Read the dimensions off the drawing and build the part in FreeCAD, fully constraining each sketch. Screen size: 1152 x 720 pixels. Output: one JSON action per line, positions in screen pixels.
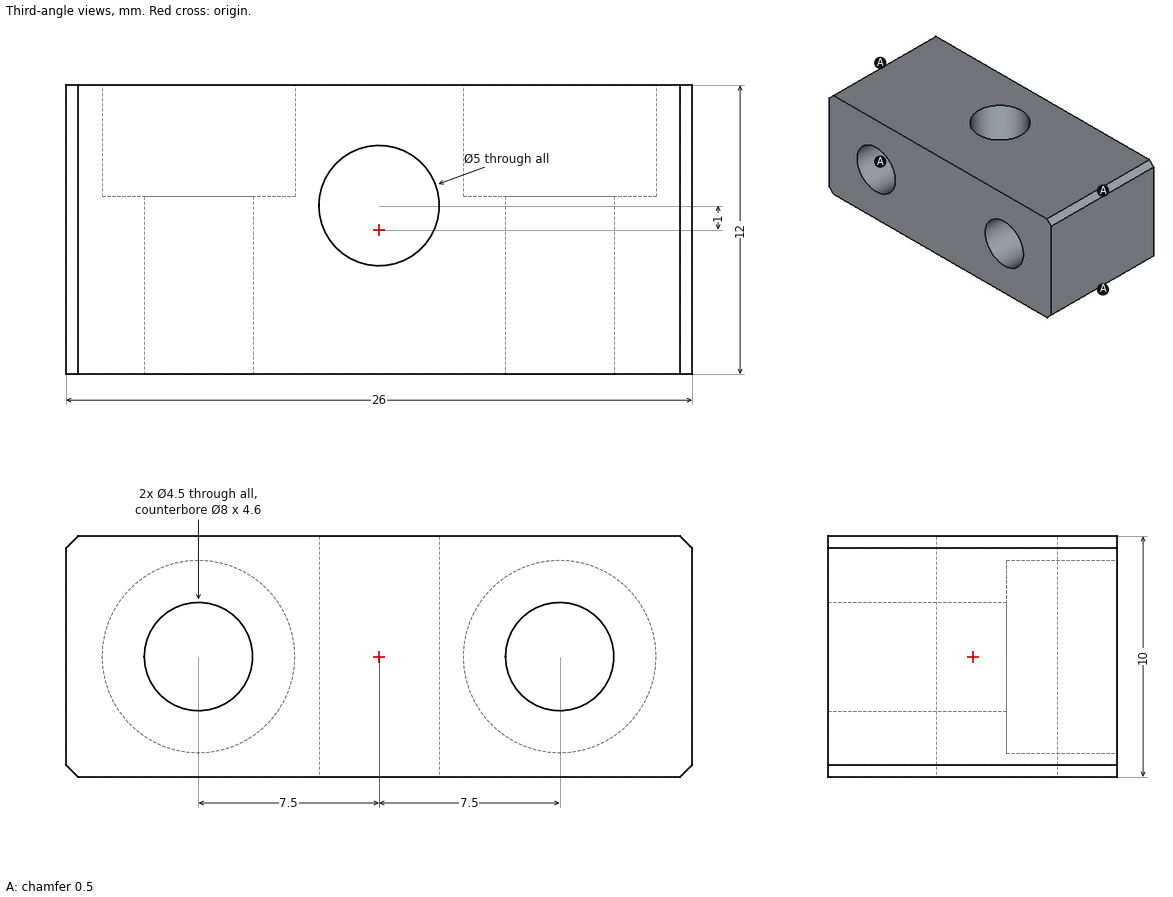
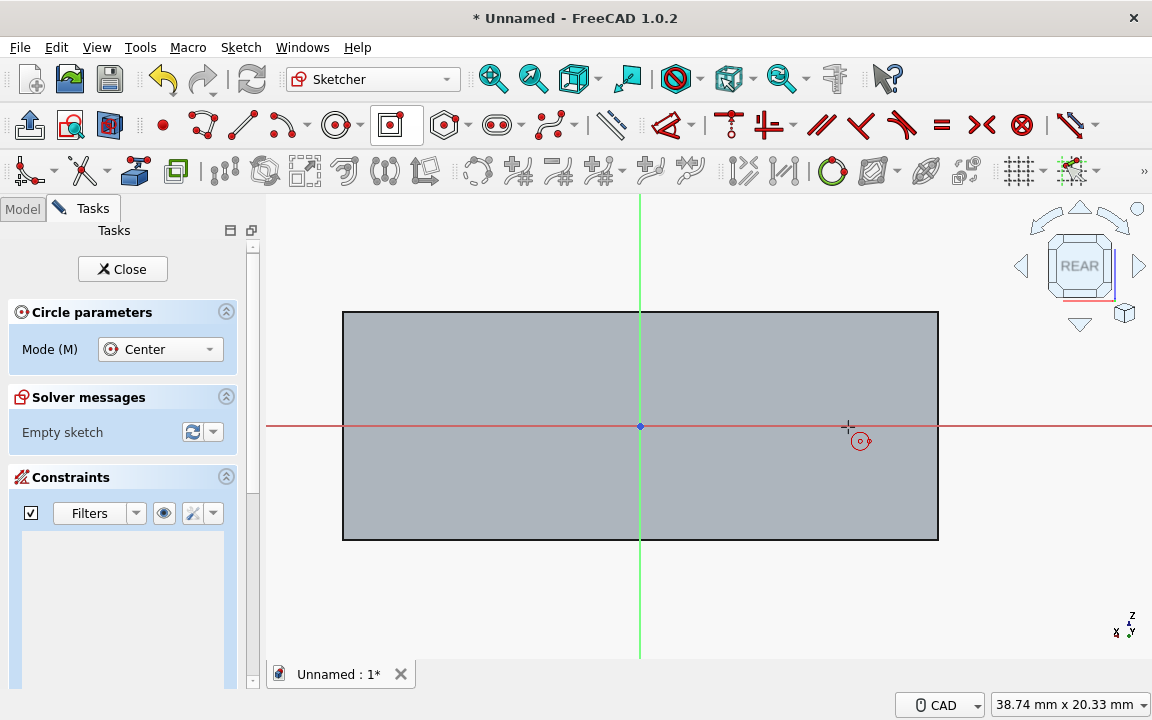
{"action": "left_click", "coordinate": [812, 426]}
{"action": "left_click", "coordinate": [848, 390]}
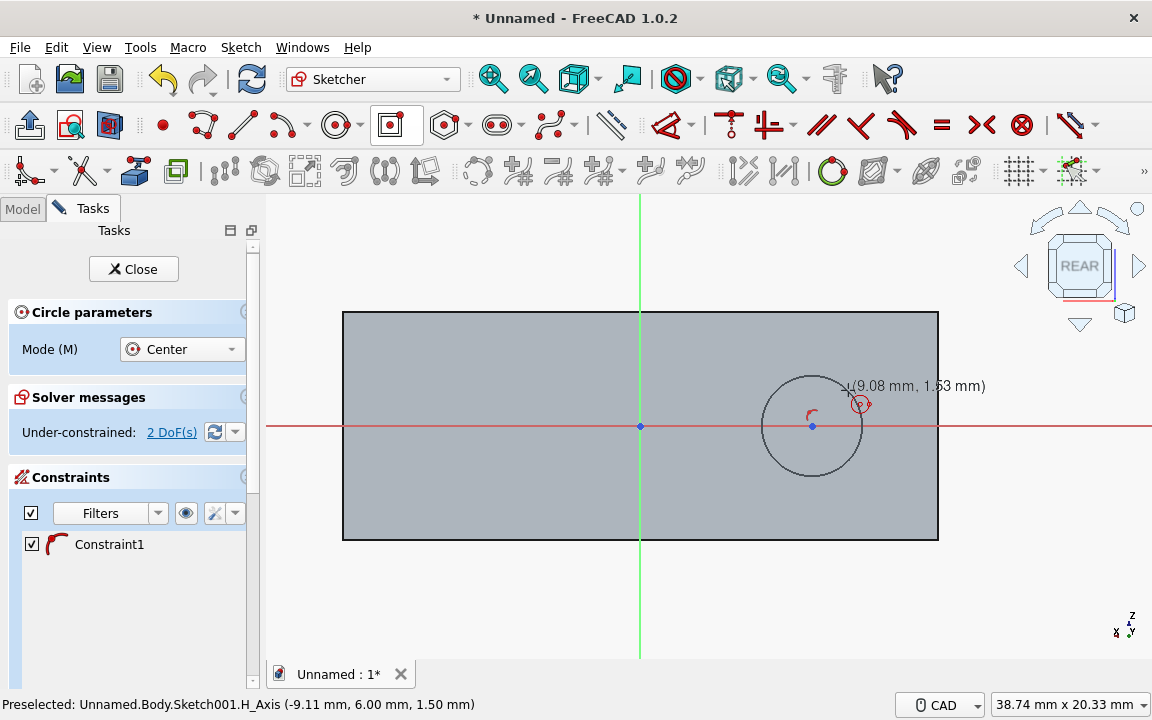
{"action": "left_click", "coordinate": [469, 426]}
{"action": "left_click", "coordinate": [505, 390]}
{"action": "key", "text": "Escape"}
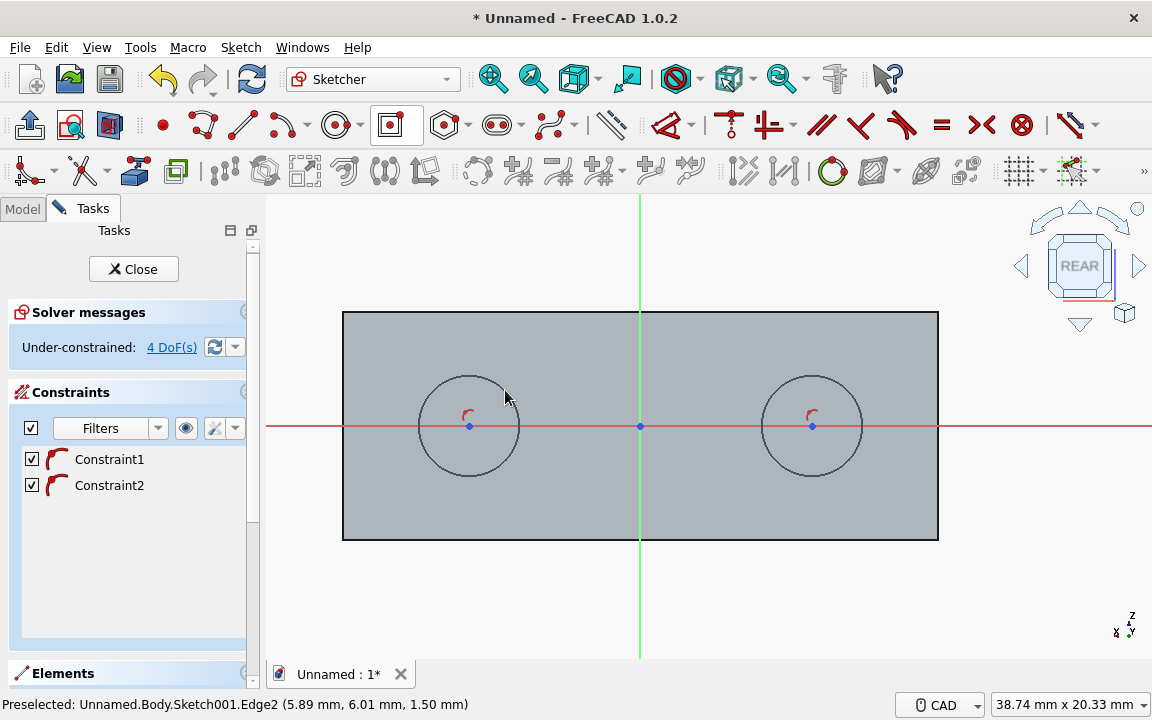
{"action": "left_click", "coordinate": [847, 390]}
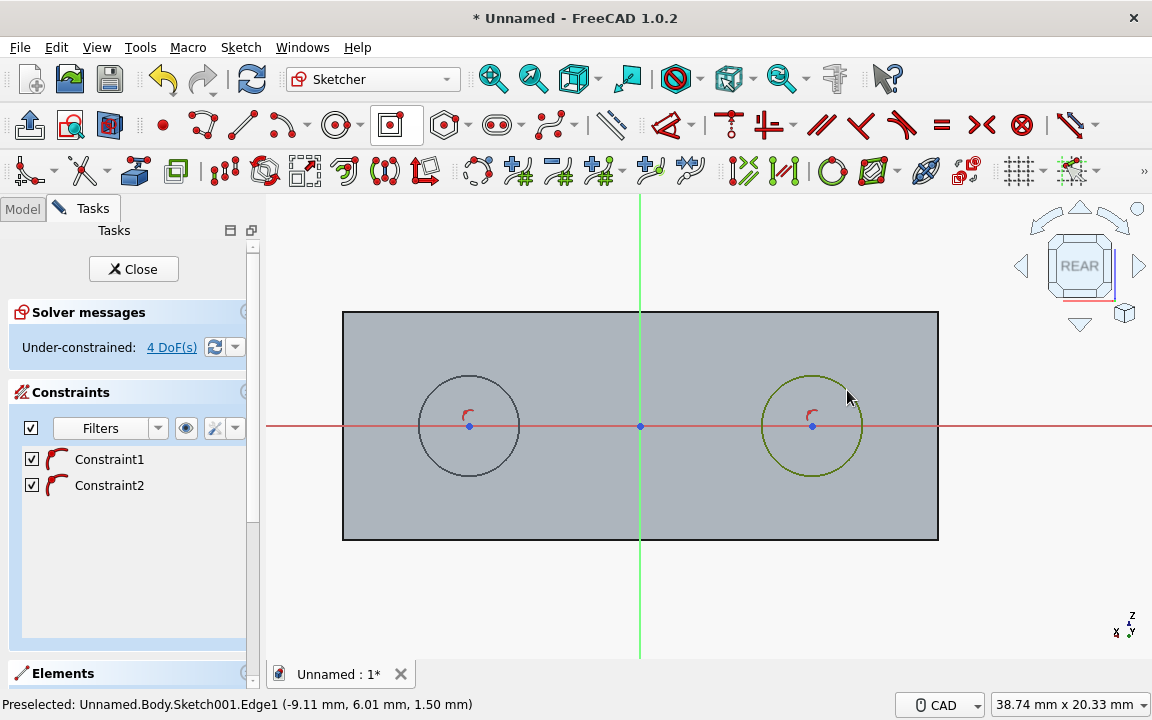
{"action": "left_click", "coordinate": [504, 390]}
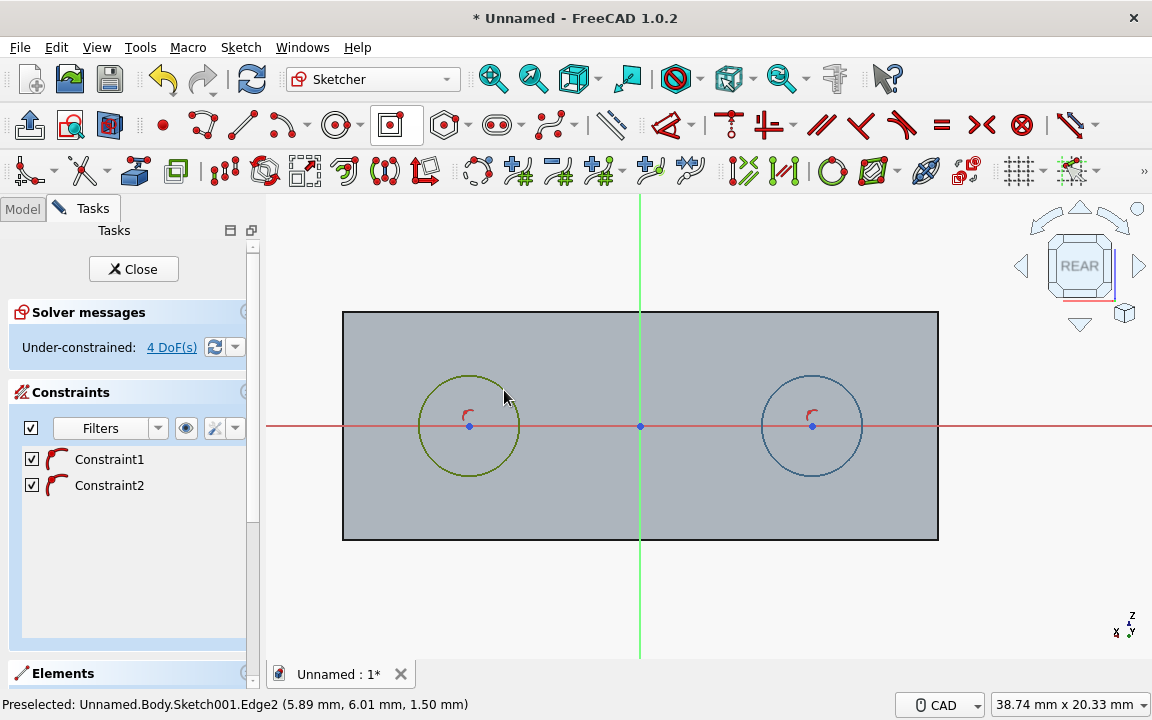
{"action": "key", "text": "e"}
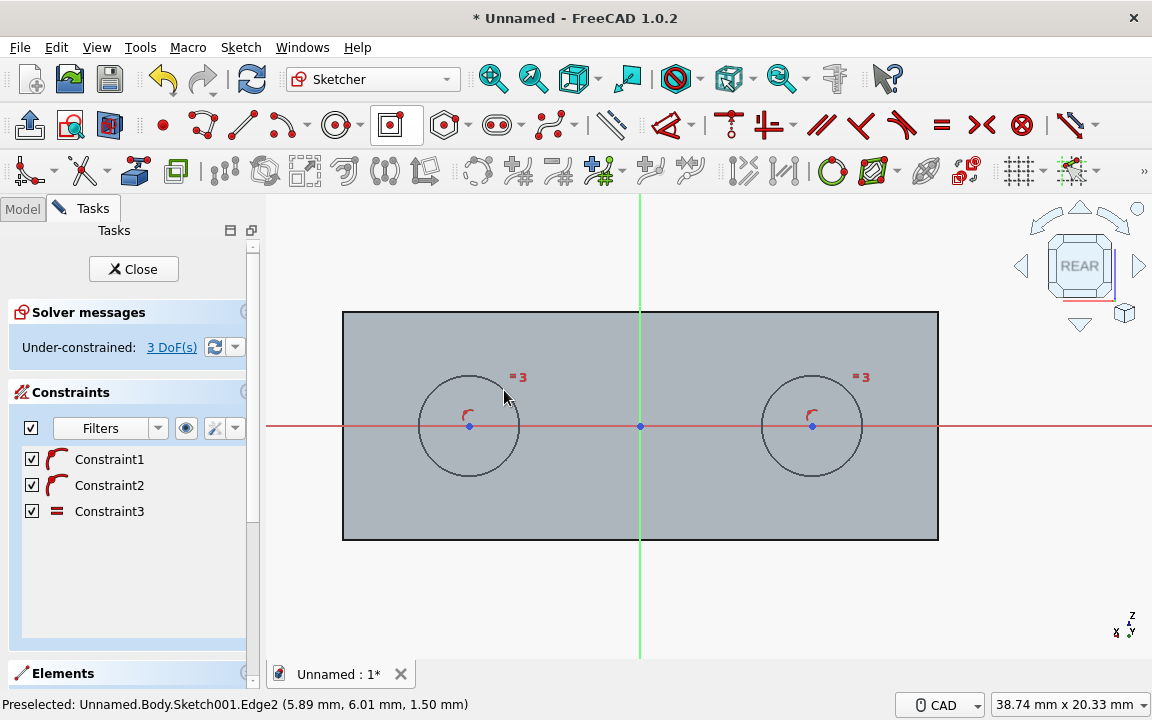
{"action": "left_click", "coordinate": [847, 390]}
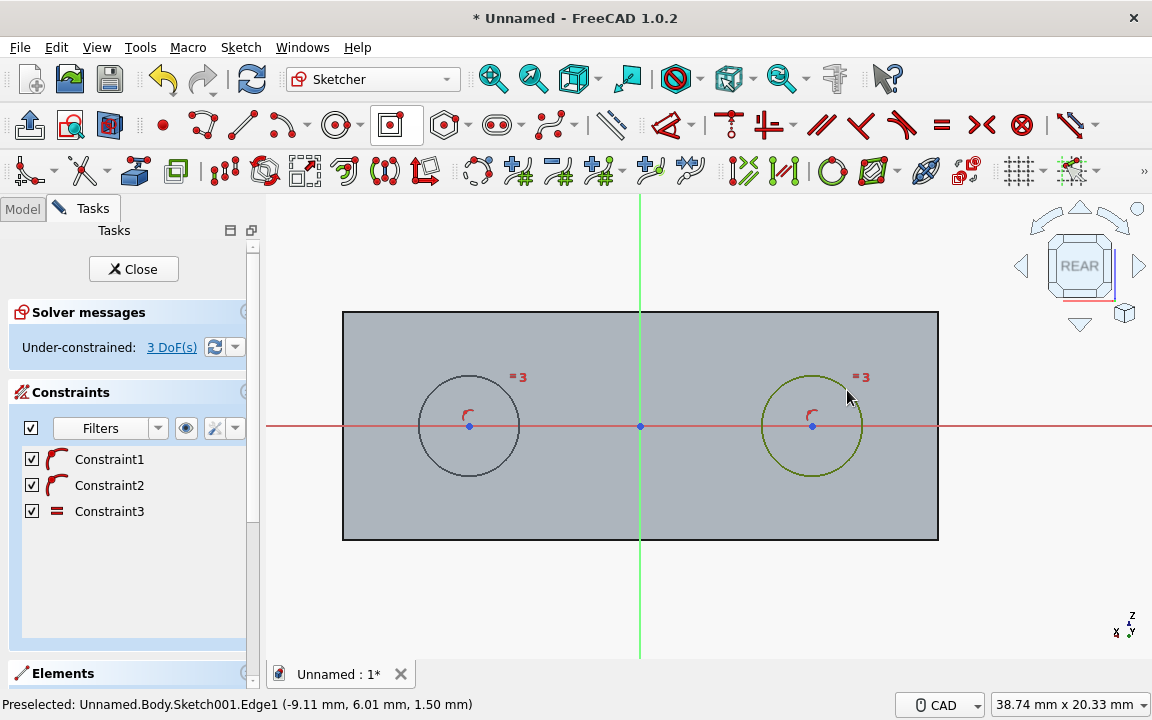
{"action": "key", "text": "k o"}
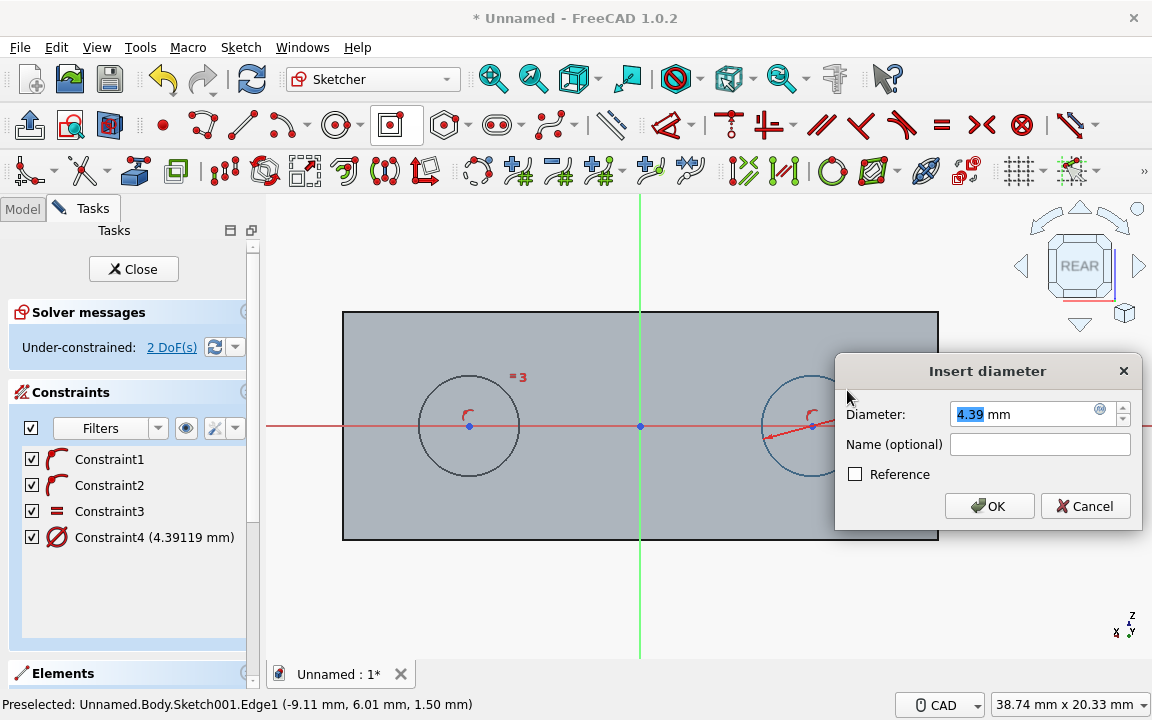
{"action": "type", "text": "4.5"}
{"action": "key", "text": "Return"}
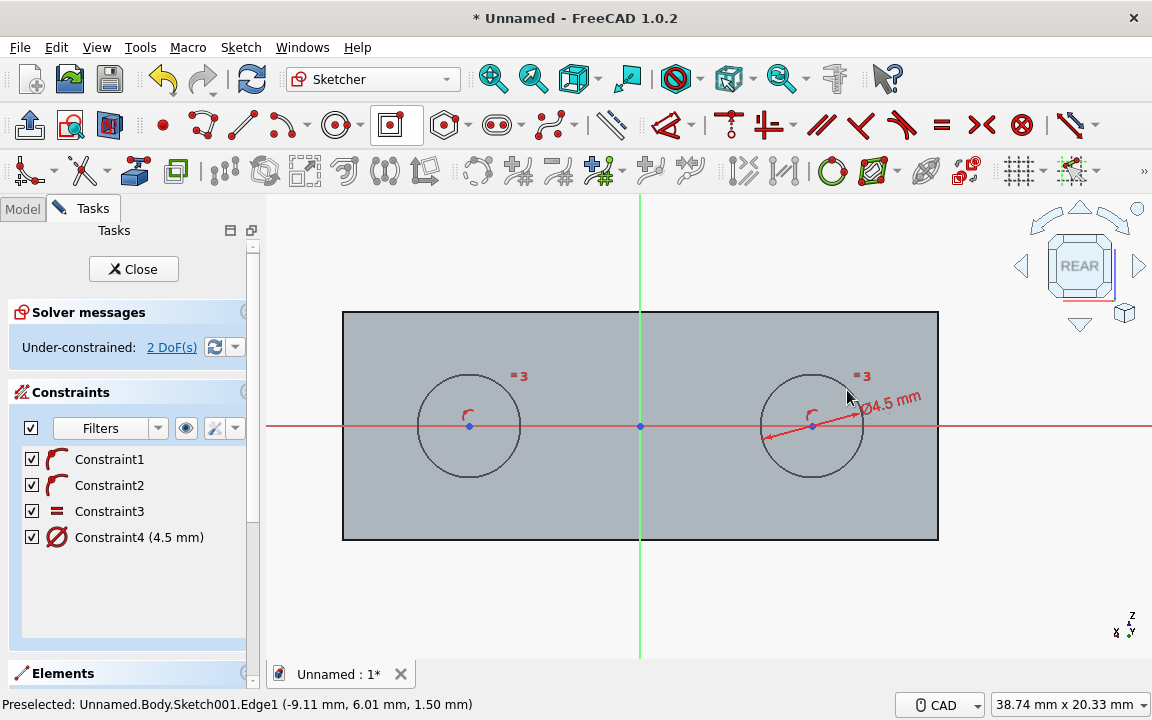
{"action": "left_click", "coordinate": [812, 426]}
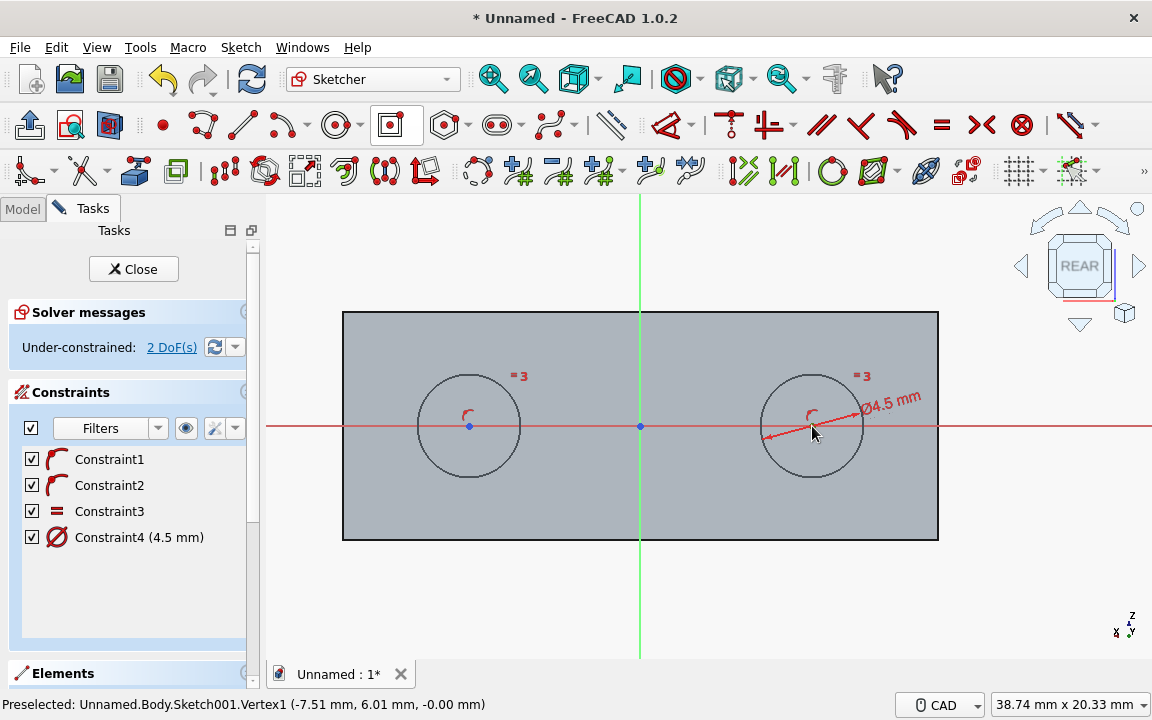
{"action": "key", "text": "l"}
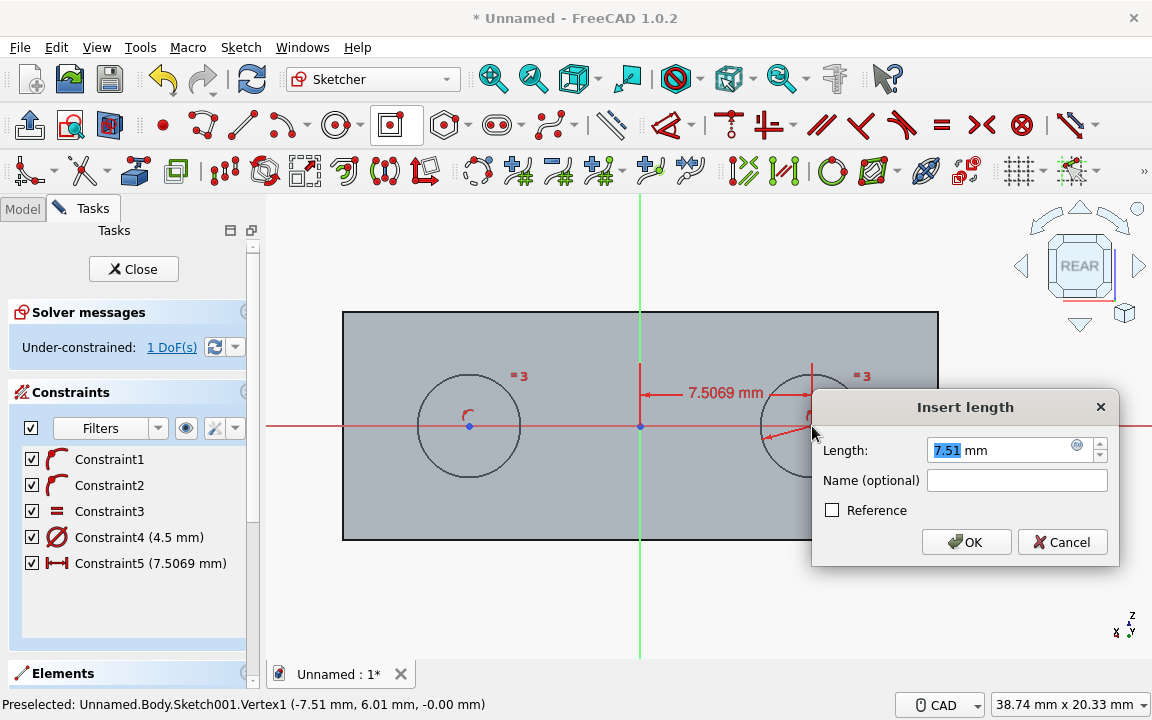
{"action": "type", "text": "7.5"}
{"action": "key", "text": "Return"}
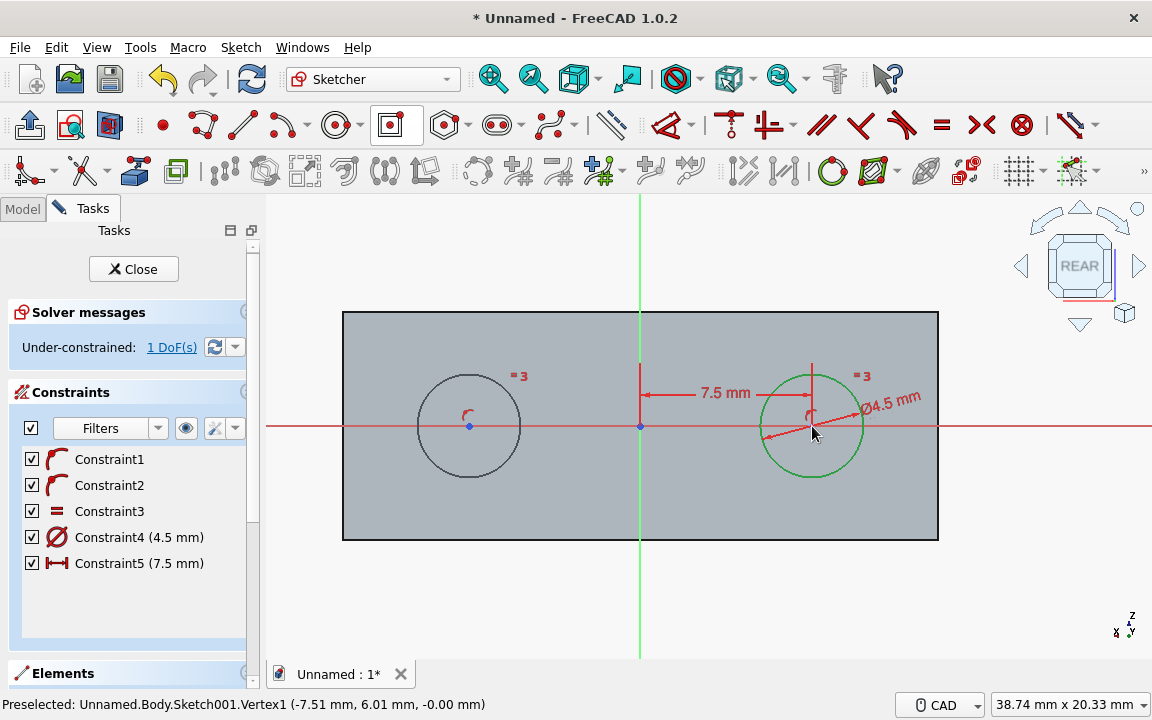
{"action": "left_click", "coordinate": [469, 426]}